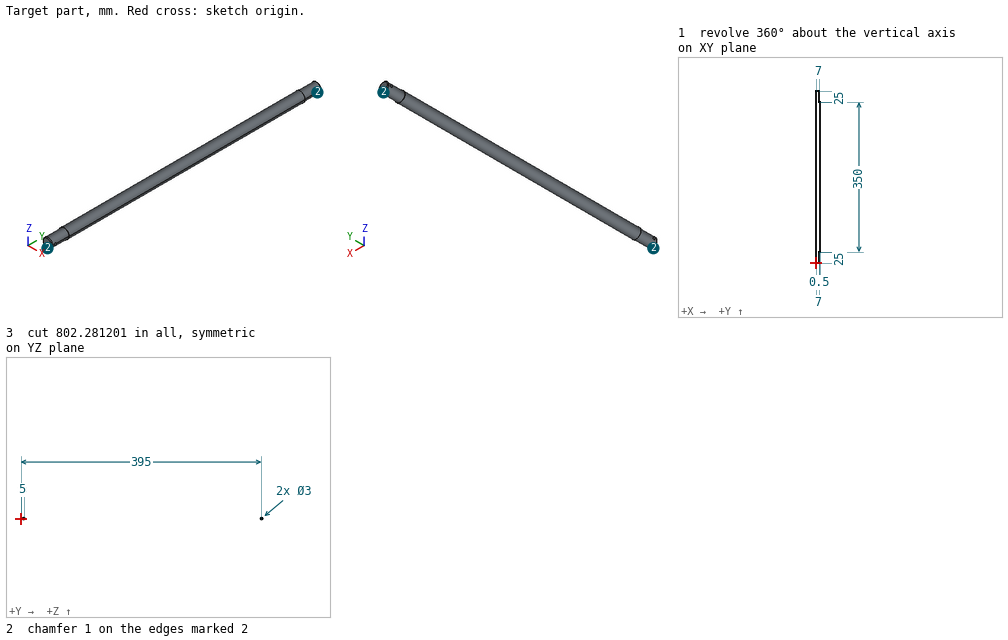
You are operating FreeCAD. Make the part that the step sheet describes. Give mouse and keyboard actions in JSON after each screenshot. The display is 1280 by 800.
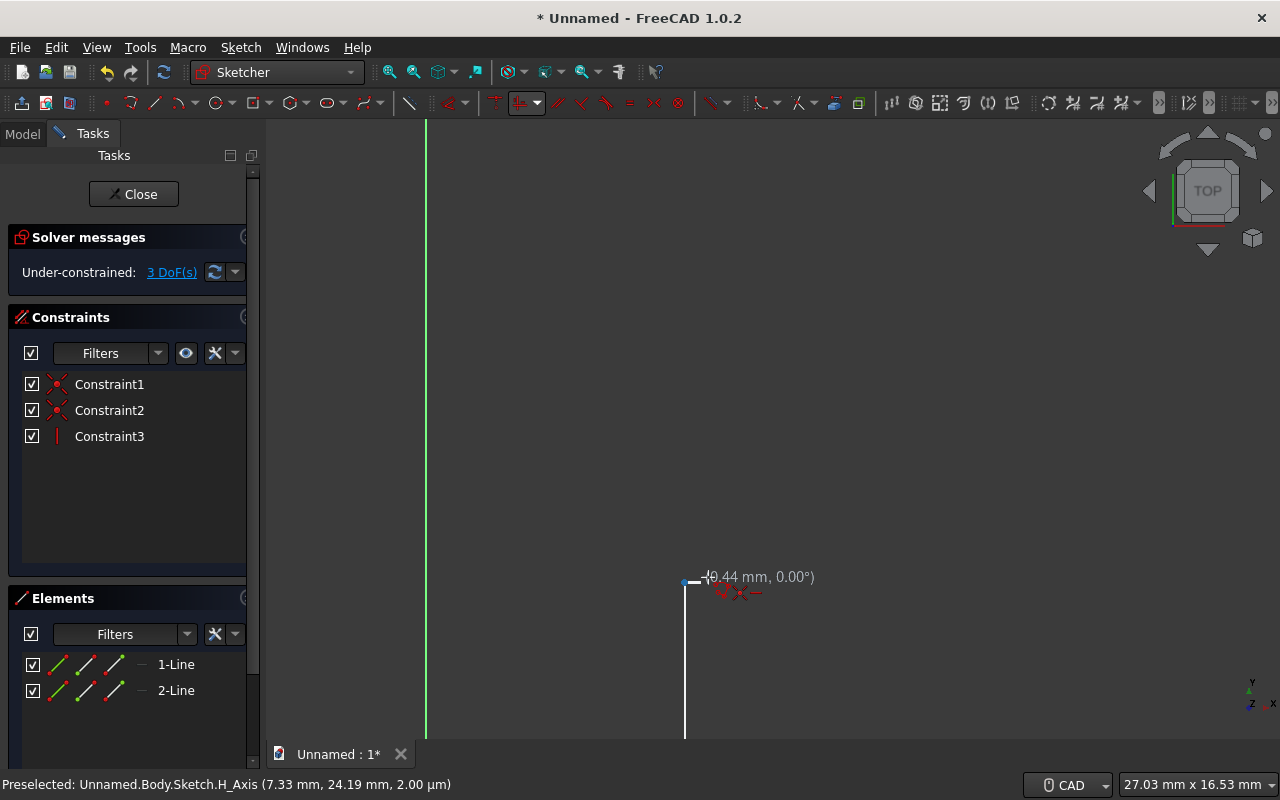
{"action": "left_click", "coordinate": [708, 566]}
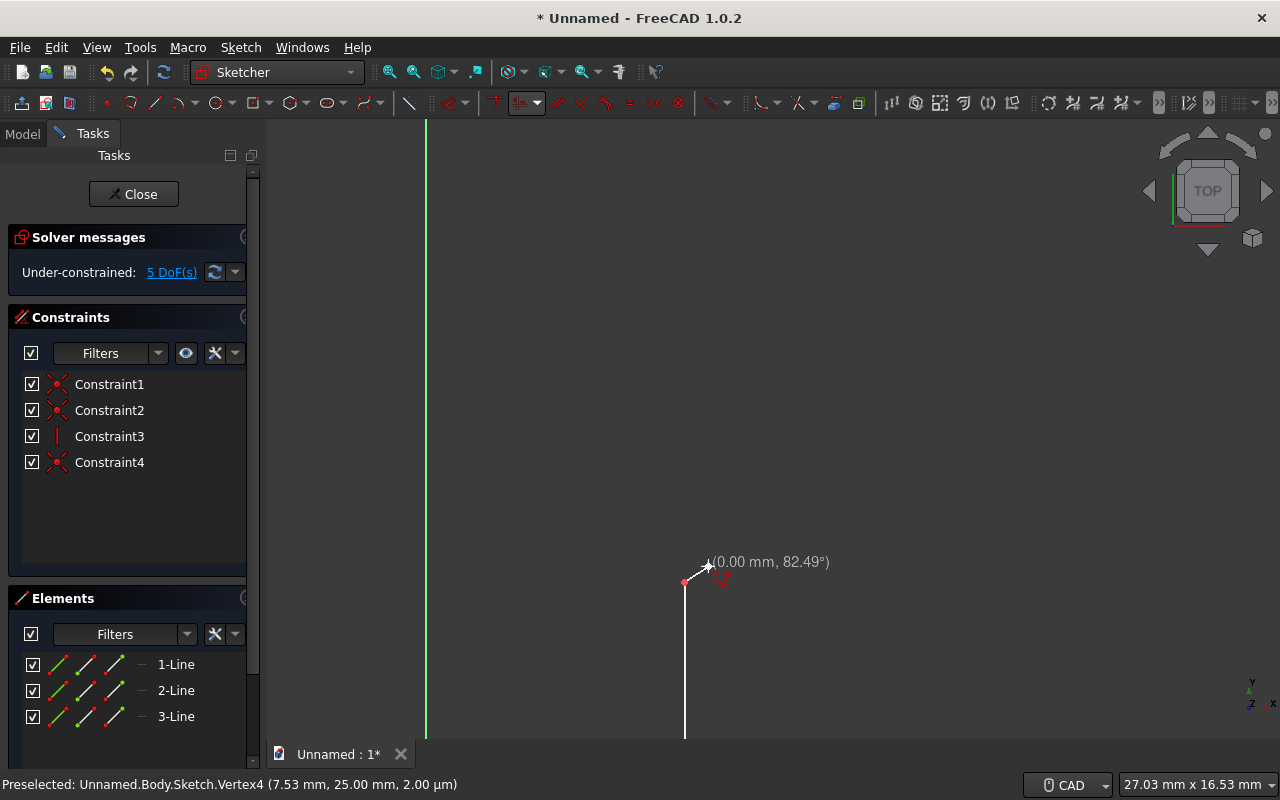
{"action": "scroll", "coordinate": [709, 651], "scroll_direction": "down", "scroll_amount": 17}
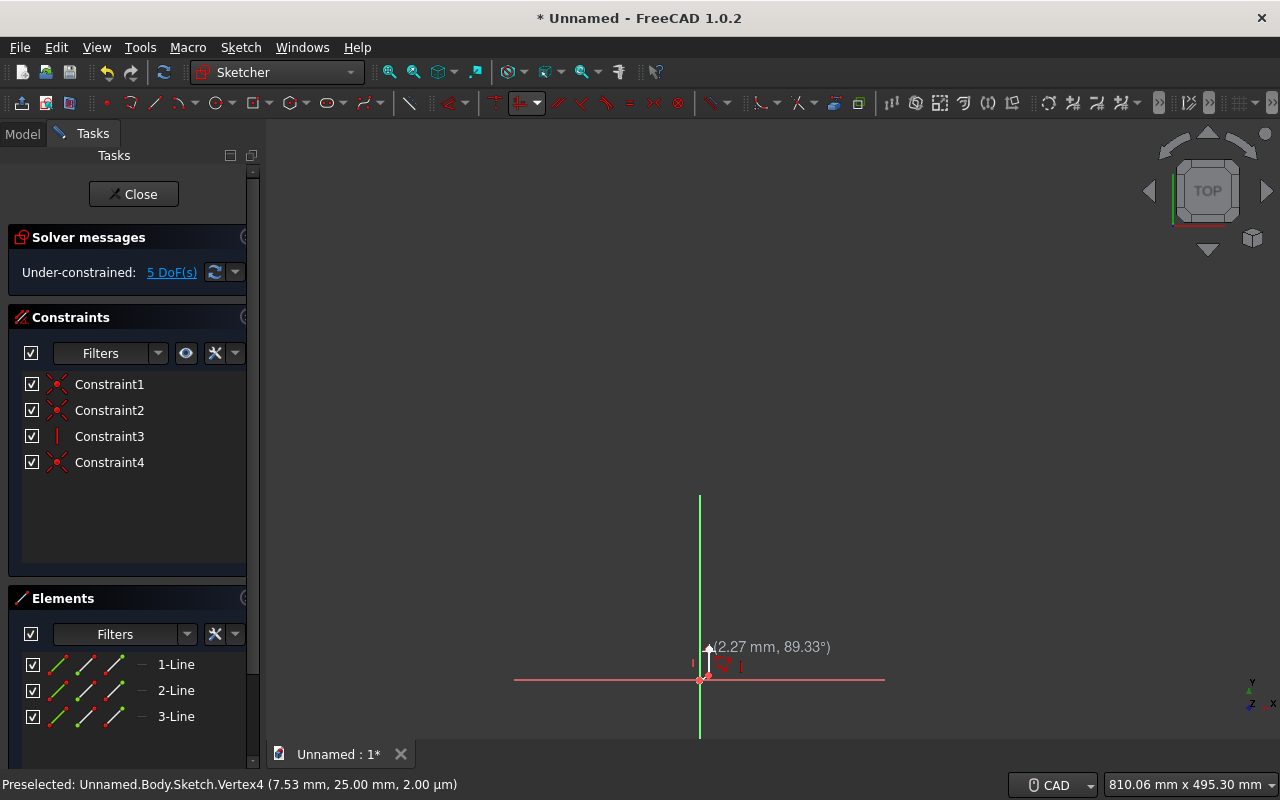
{"action": "scroll", "coordinate": [709, 211], "scroll_direction": "up", "scroll_amount": 3}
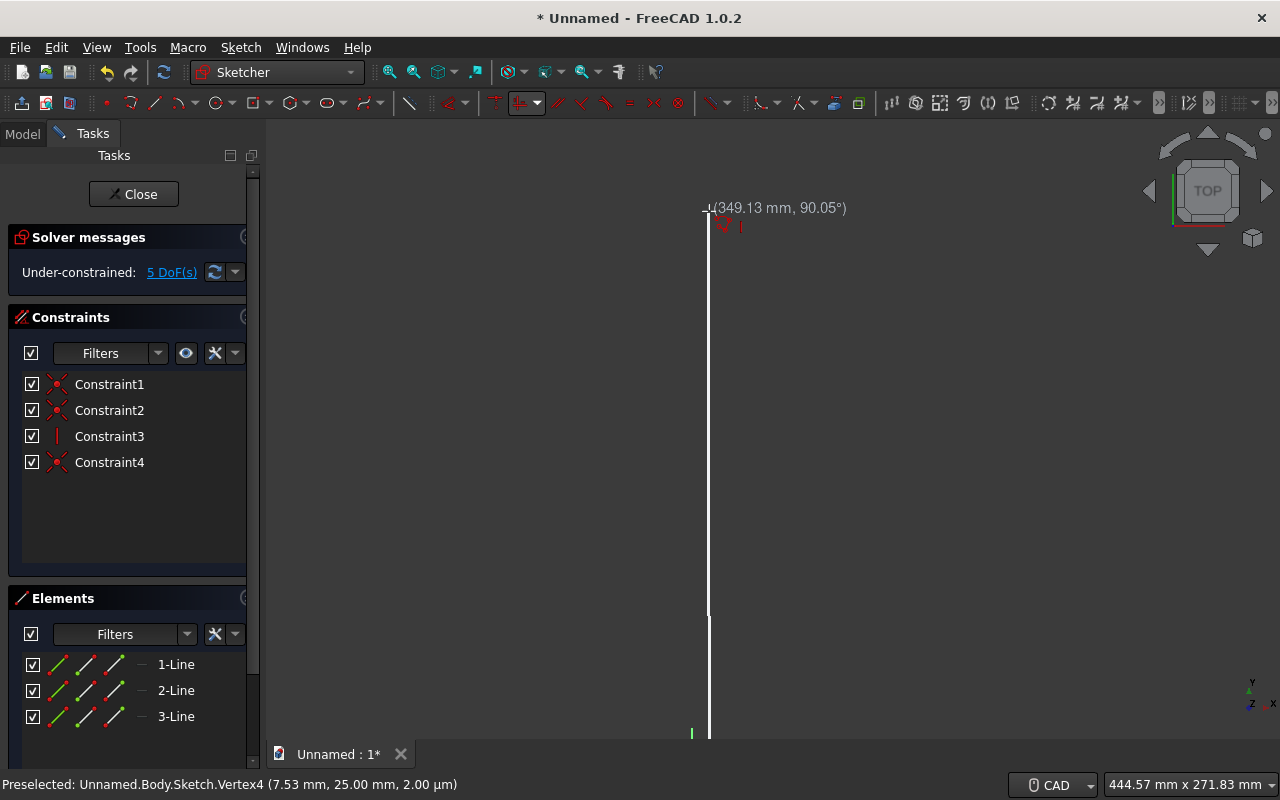
{"action": "left_click", "coordinate": [709, 211]}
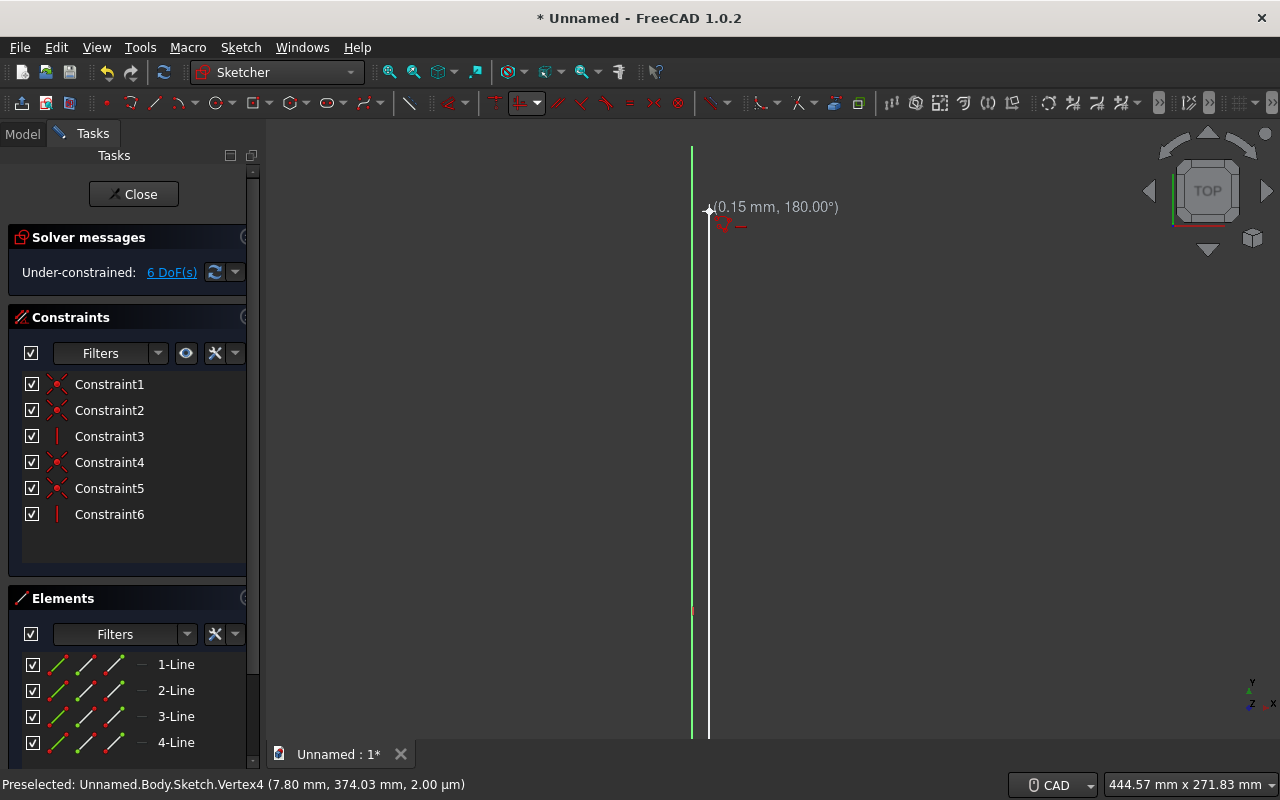
{"action": "scroll", "coordinate": [708, 211], "scroll_direction": "up", "scroll_amount": 14}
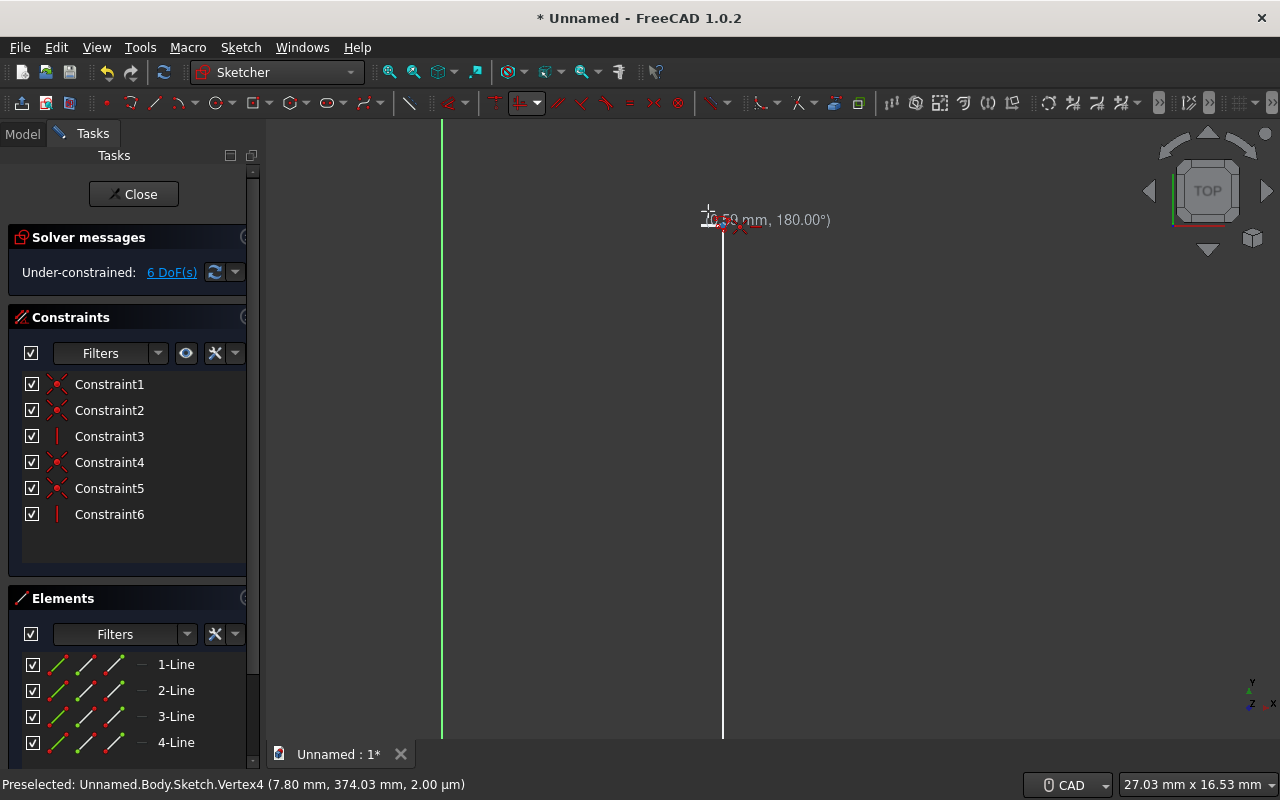
{"action": "left_click", "coordinate": [704, 209]}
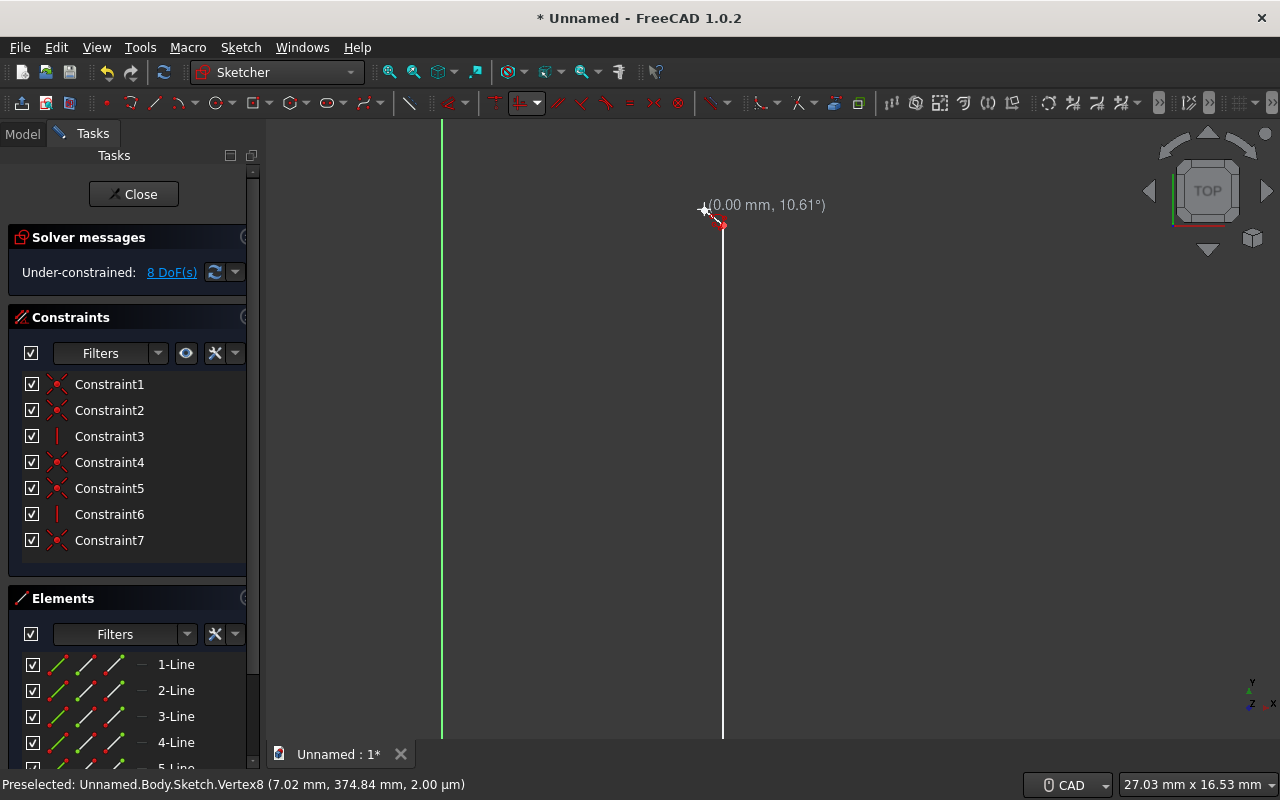
{"action": "scroll", "coordinate": [709, 210], "scroll_direction": "down", "scroll_amount": 17}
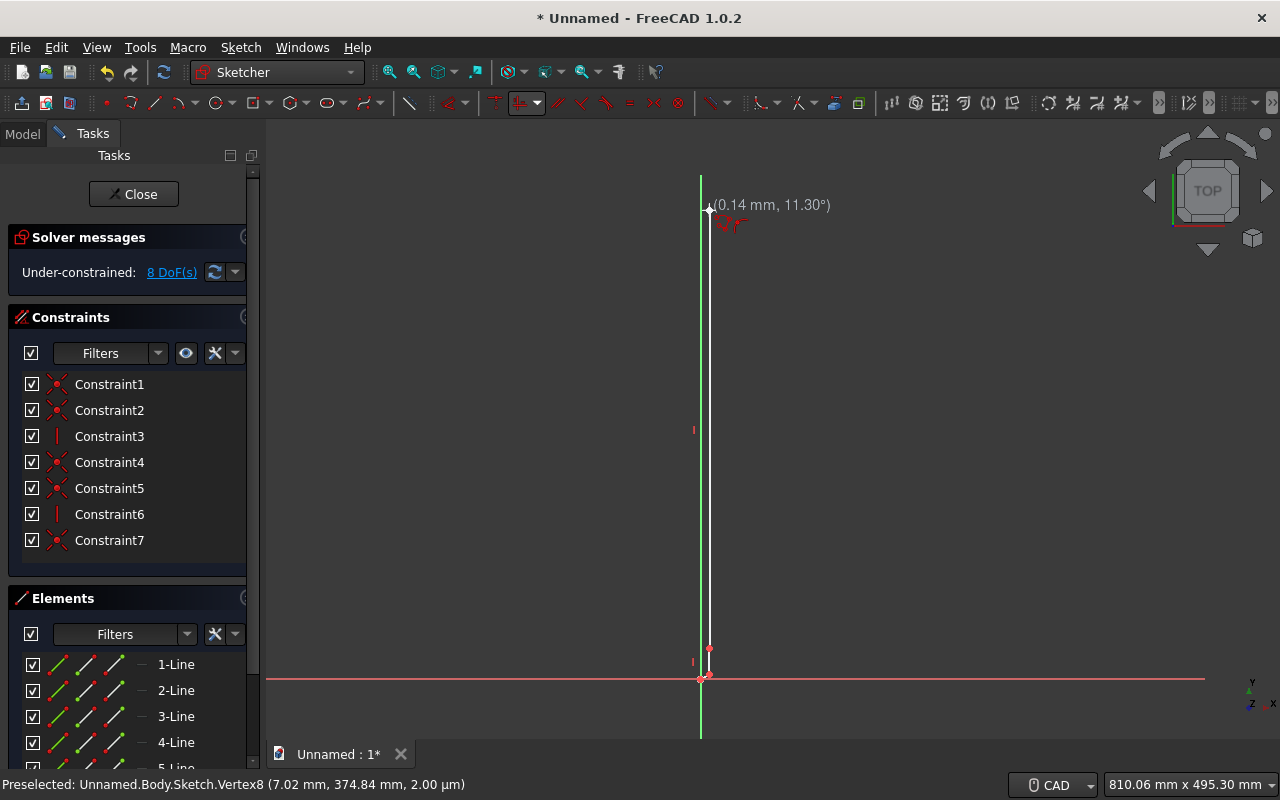
{"action": "scroll", "coordinate": [709, 179], "scroll_direction": "up", "scroll_amount": 3}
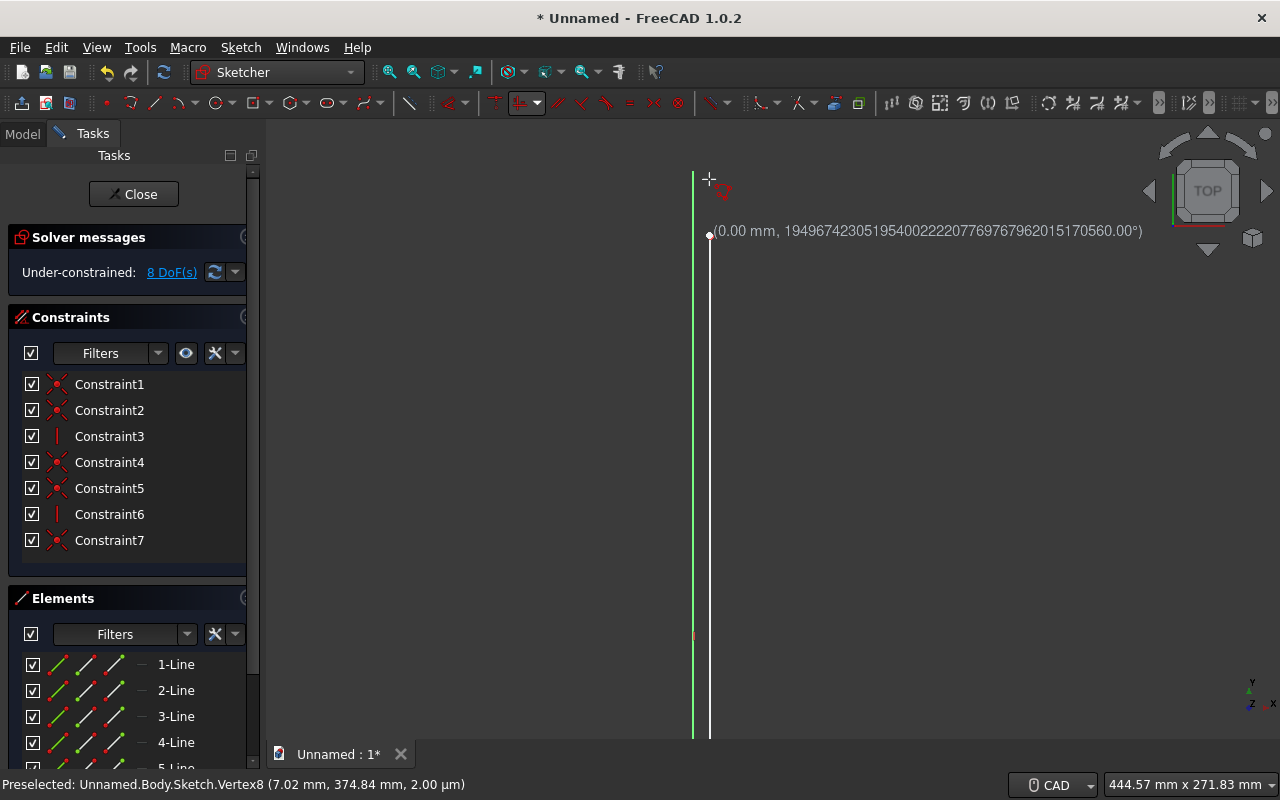
{"action": "left_click", "coordinate": [709, 178]}
{"action": "left_click", "coordinate": [702, 178]}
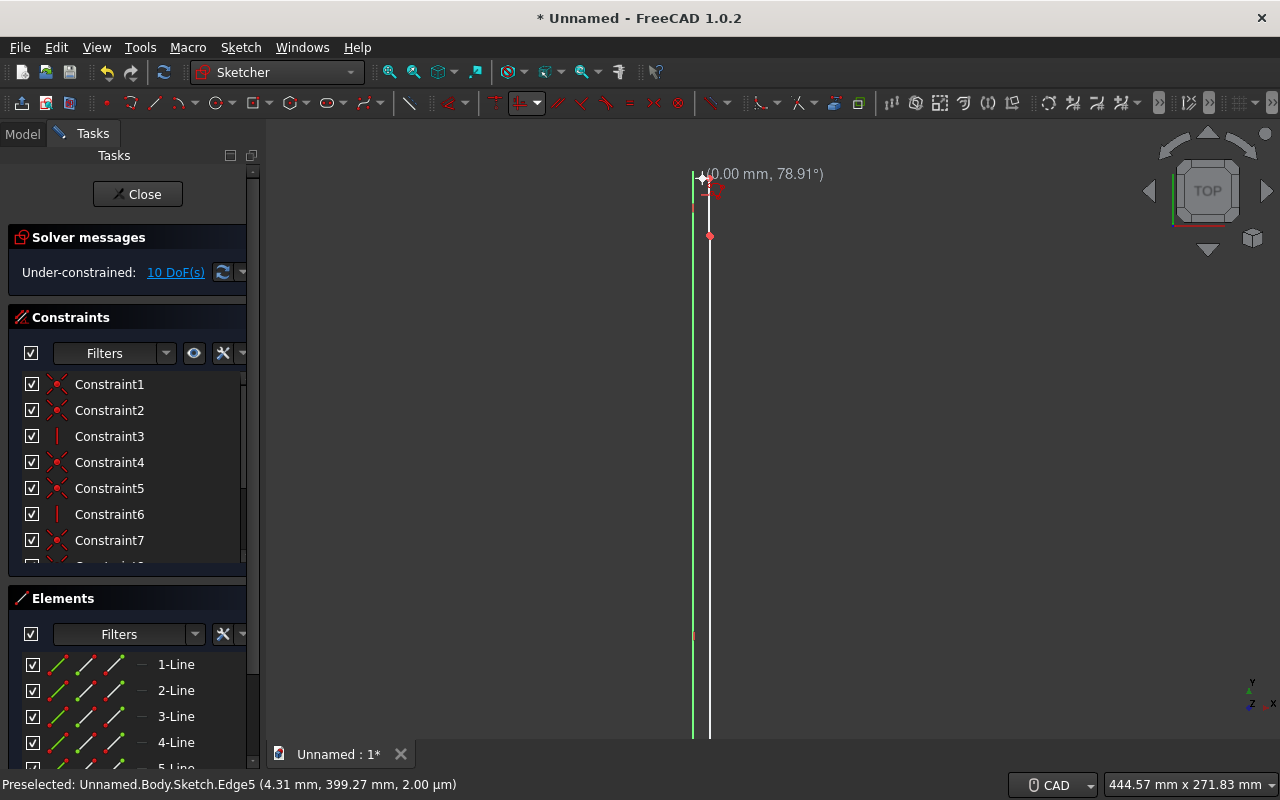
{"action": "scroll", "coordinate": [707, 261], "scroll_direction": "down", "scroll_amount": 4}